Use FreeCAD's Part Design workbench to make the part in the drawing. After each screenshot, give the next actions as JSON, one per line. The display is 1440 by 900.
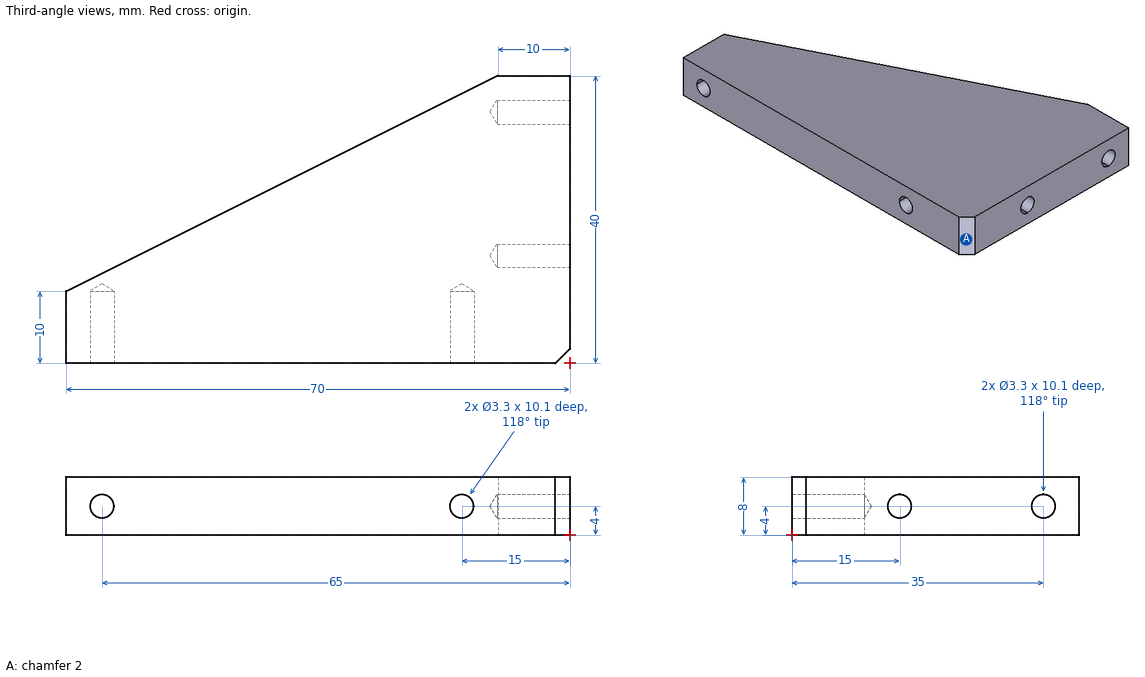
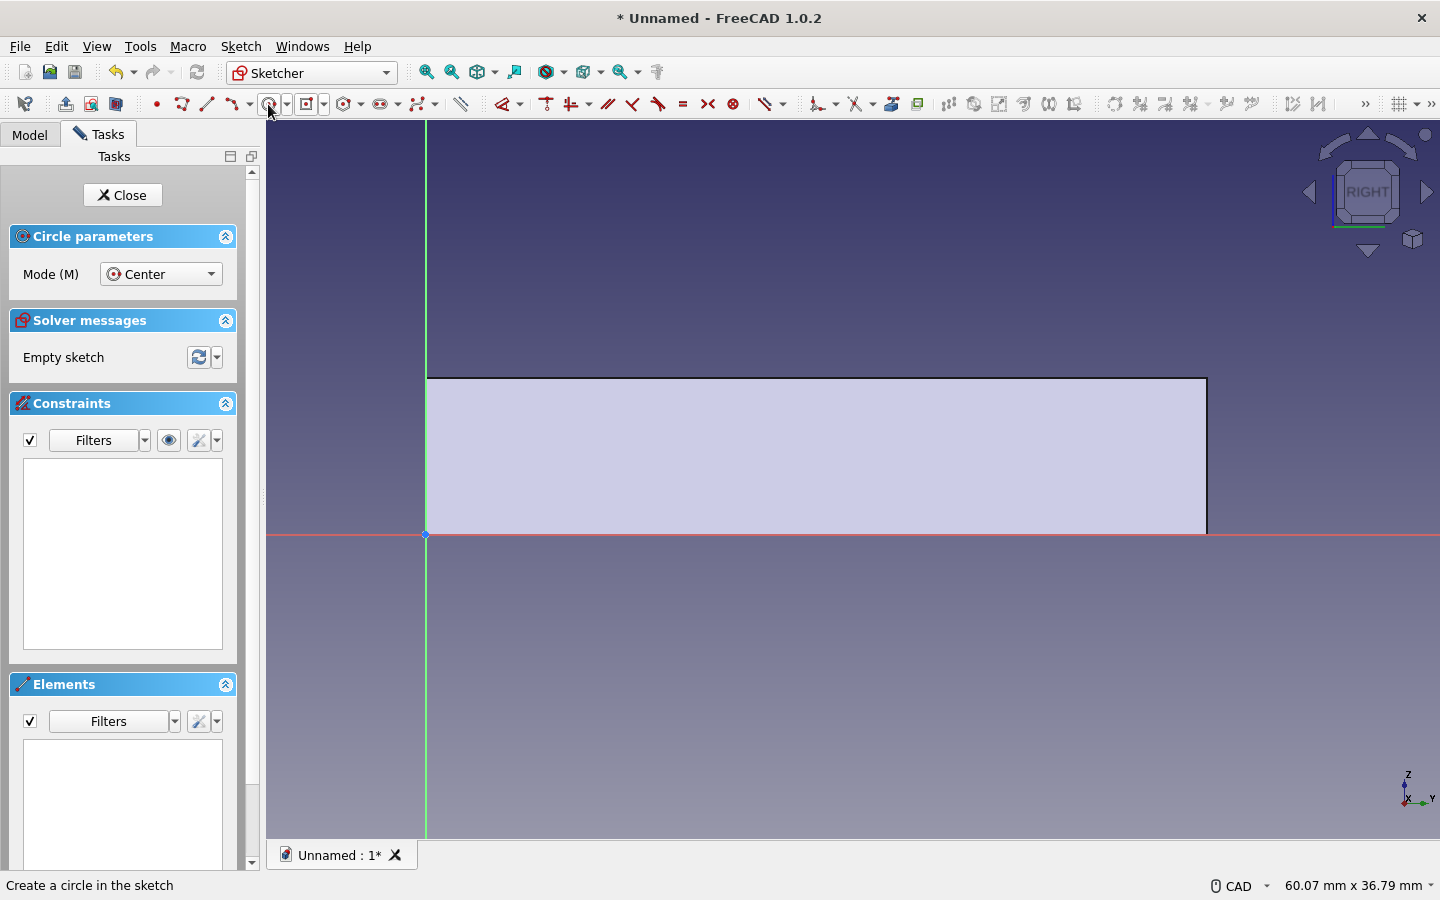
{"action": "left_click", "coordinate": [1110, 456]}
{"action": "left_click", "coordinate": [1133, 434]}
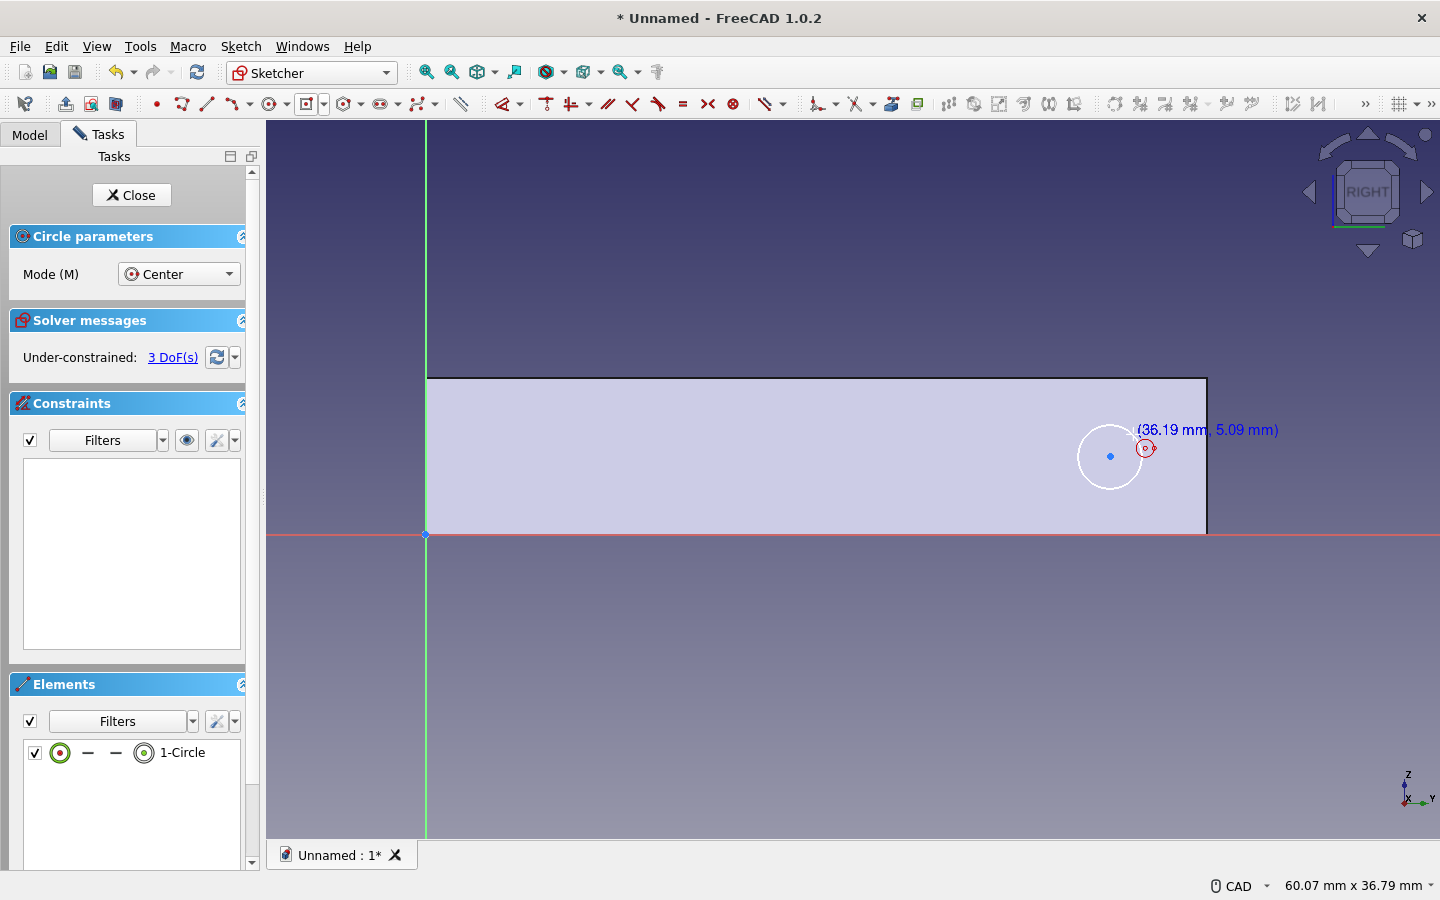
{"action": "left_click", "coordinate": [719, 456]}
{"action": "left_click", "coordinate": [742, 434]}
{"action": "key", "text": "Escape"}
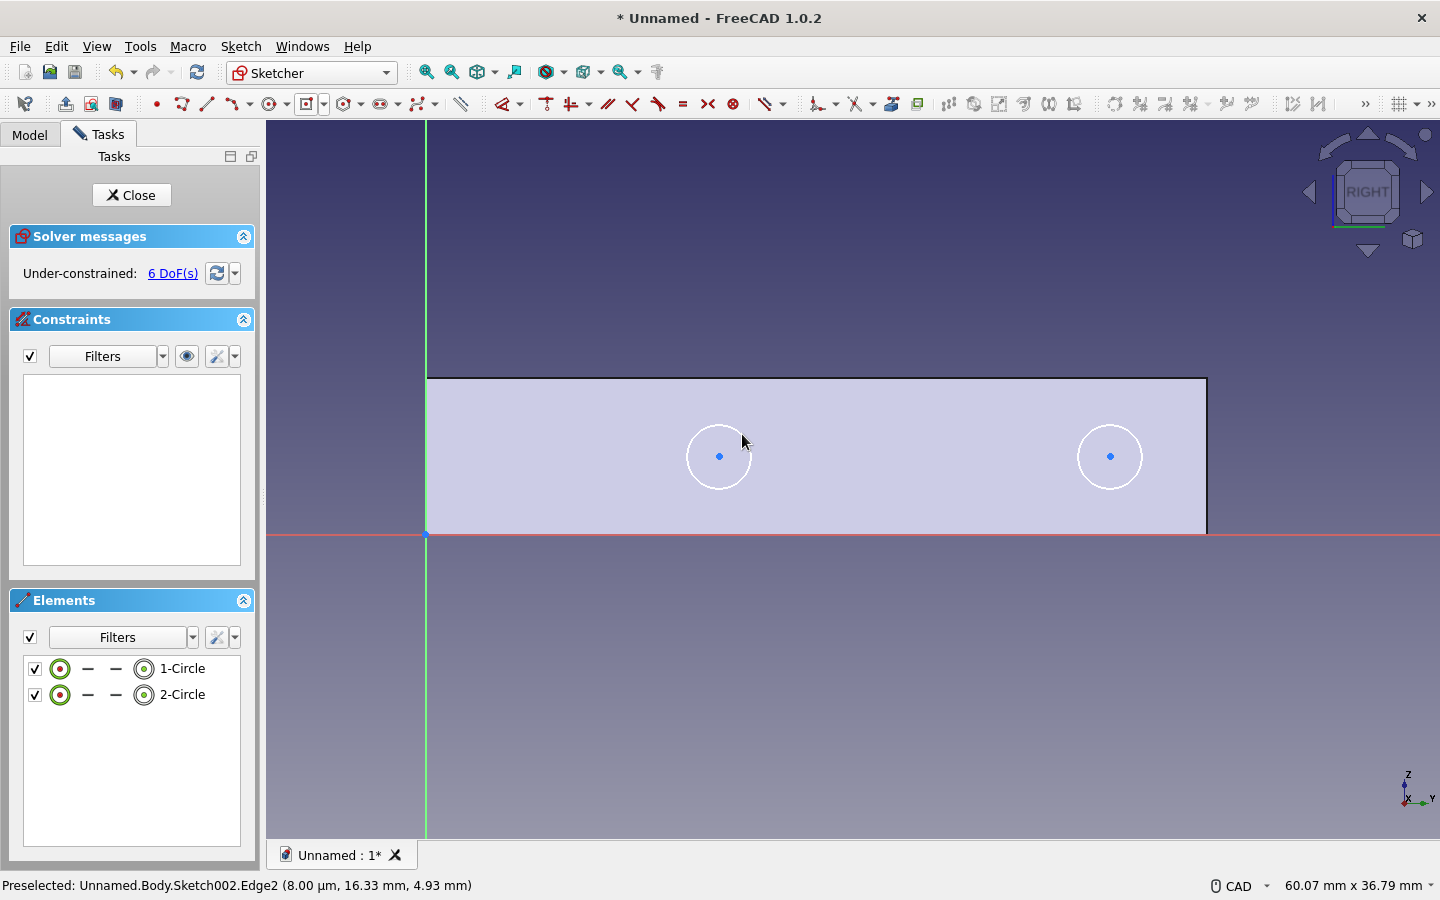
{"action": "left_click", "coordinate": [1132, 434]}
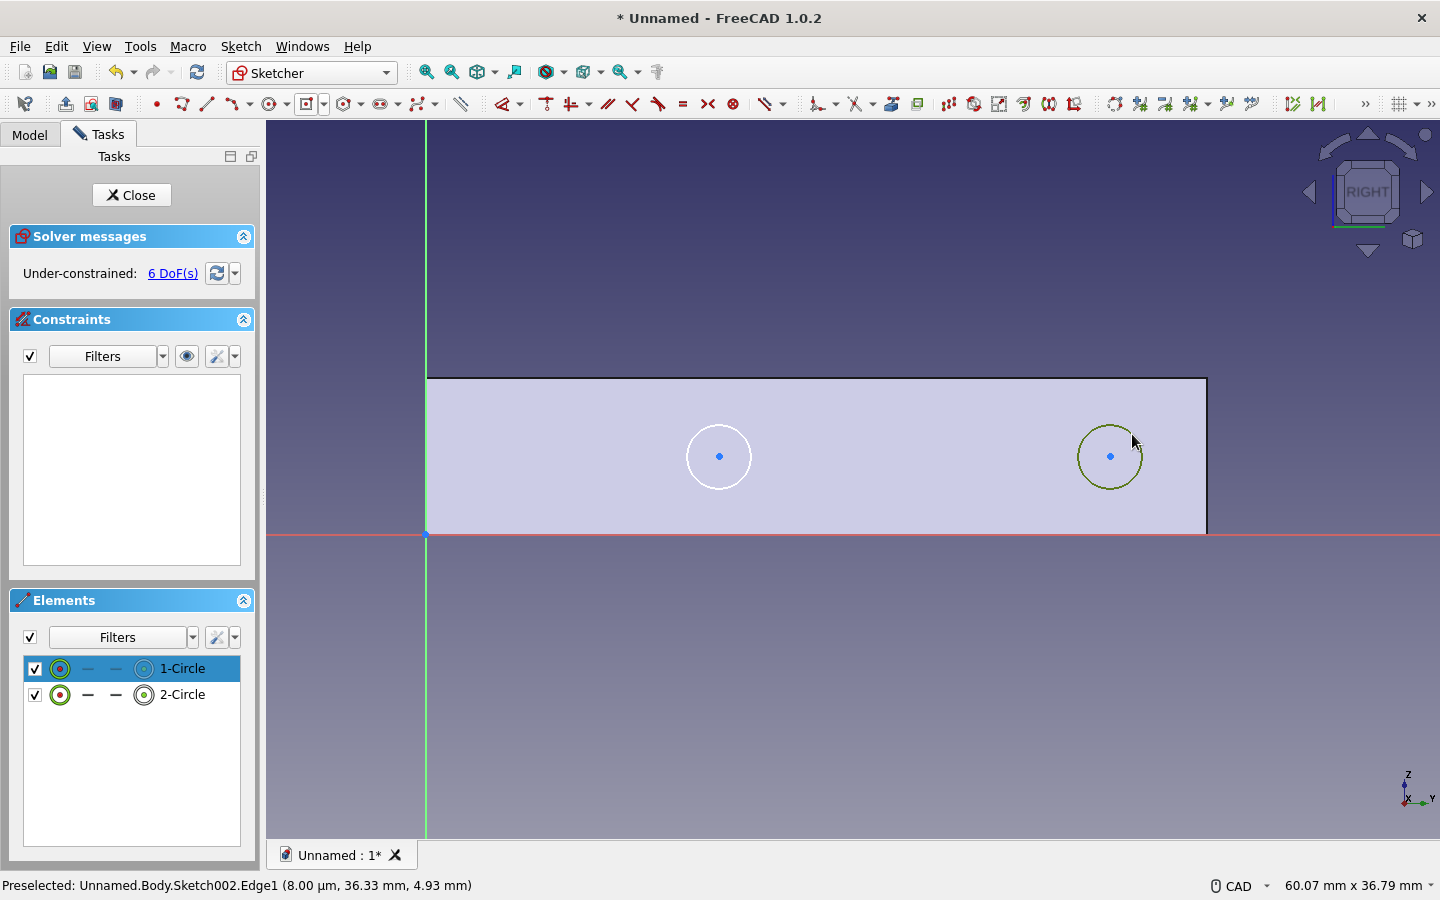
{"action": "left_click", "coordinate": [741, 434]}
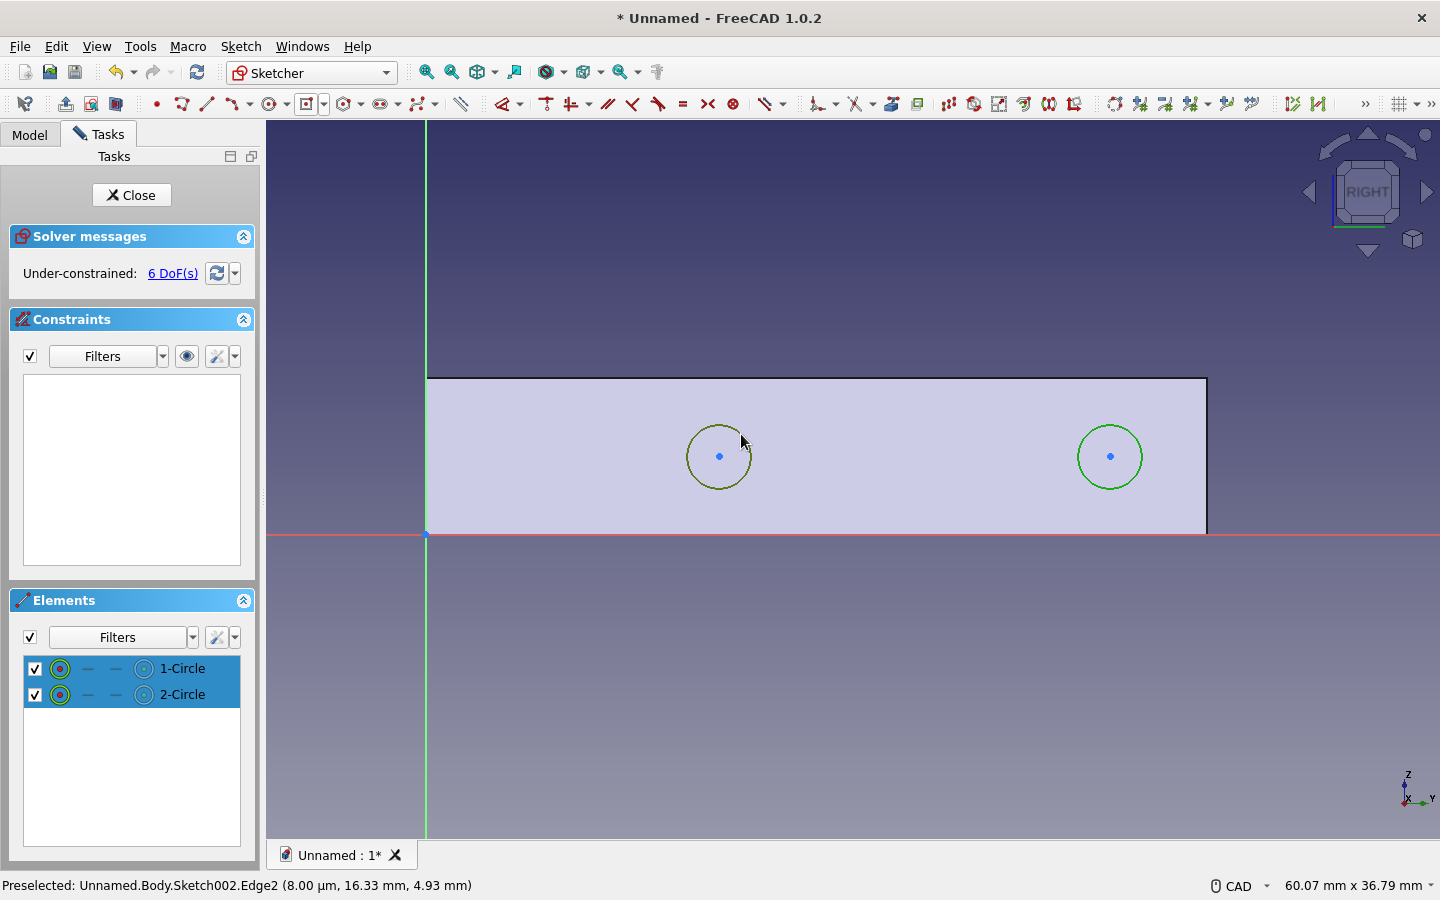
{"action": "left_click", "coordinate": [683, 104]}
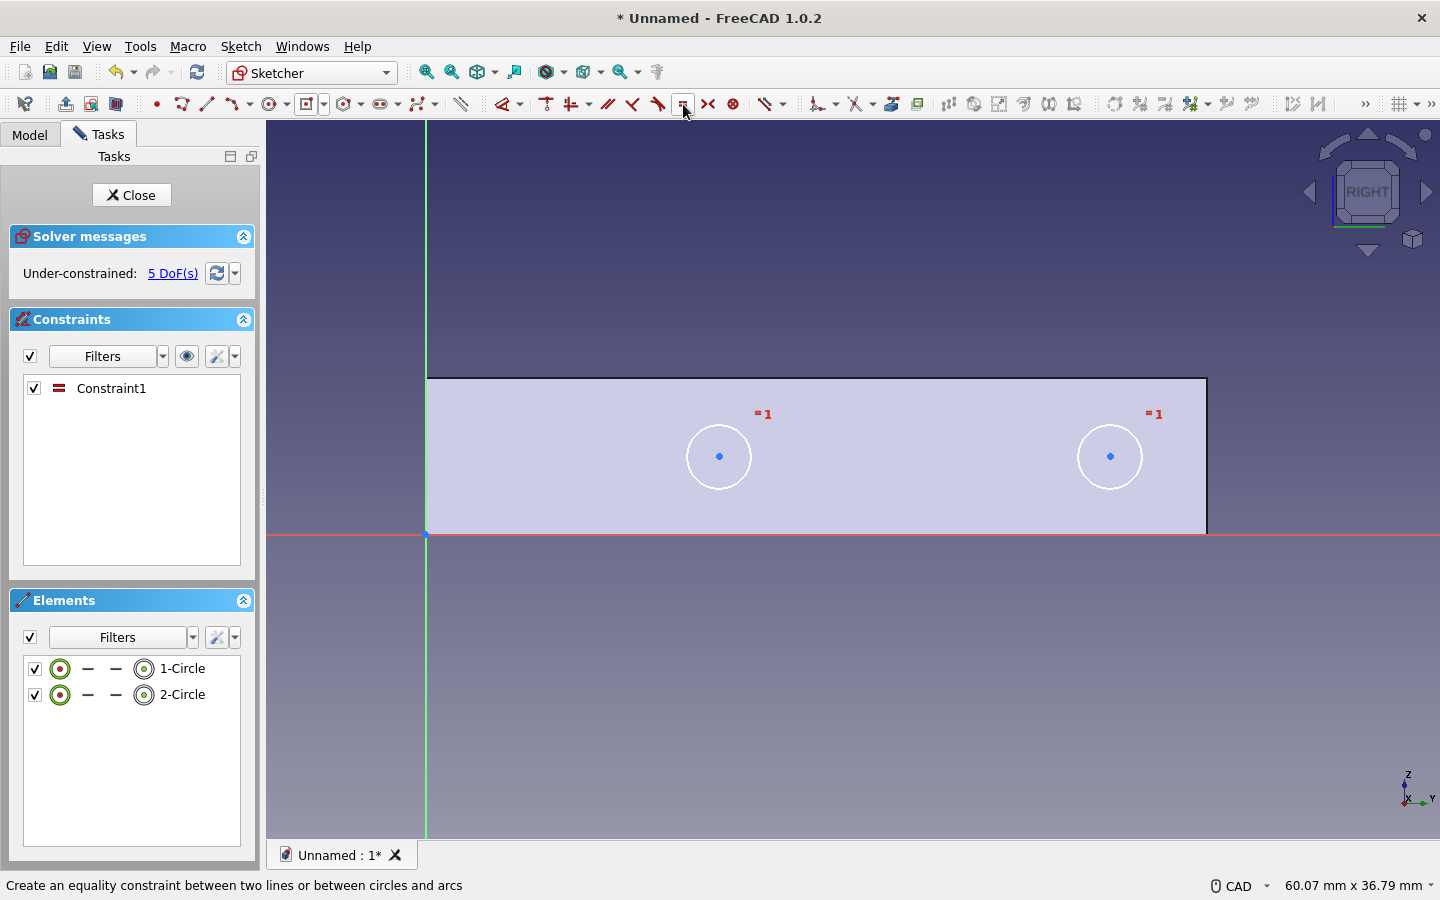
{"action": "left_click", "coordinate": [1110, 457]}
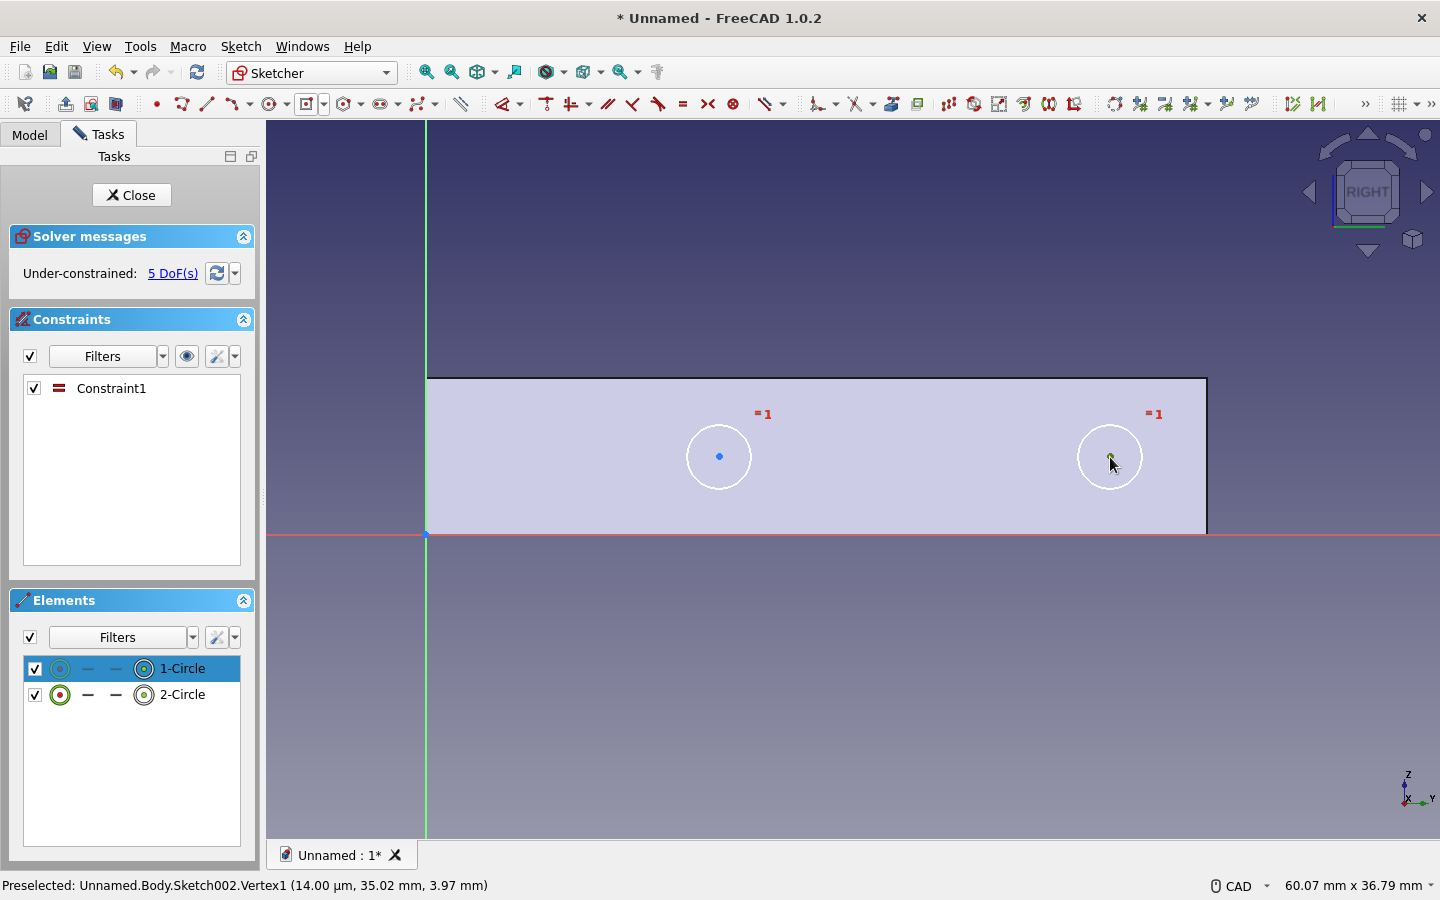
{"action": "left_click", "coordinate": [719, 457]}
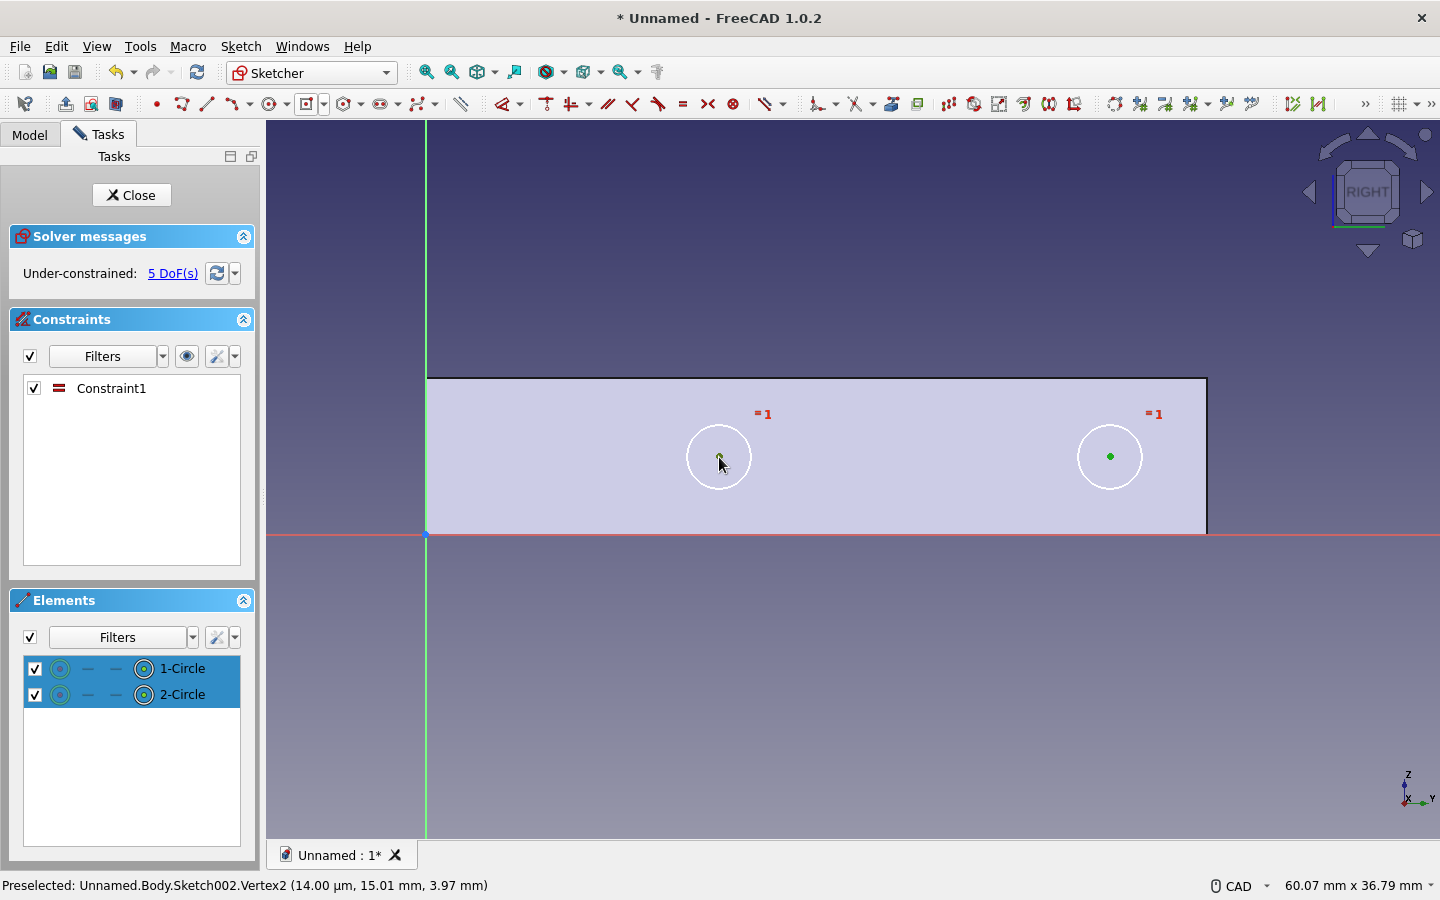
{"action": "left_click", "coordinate": [588, 104]}